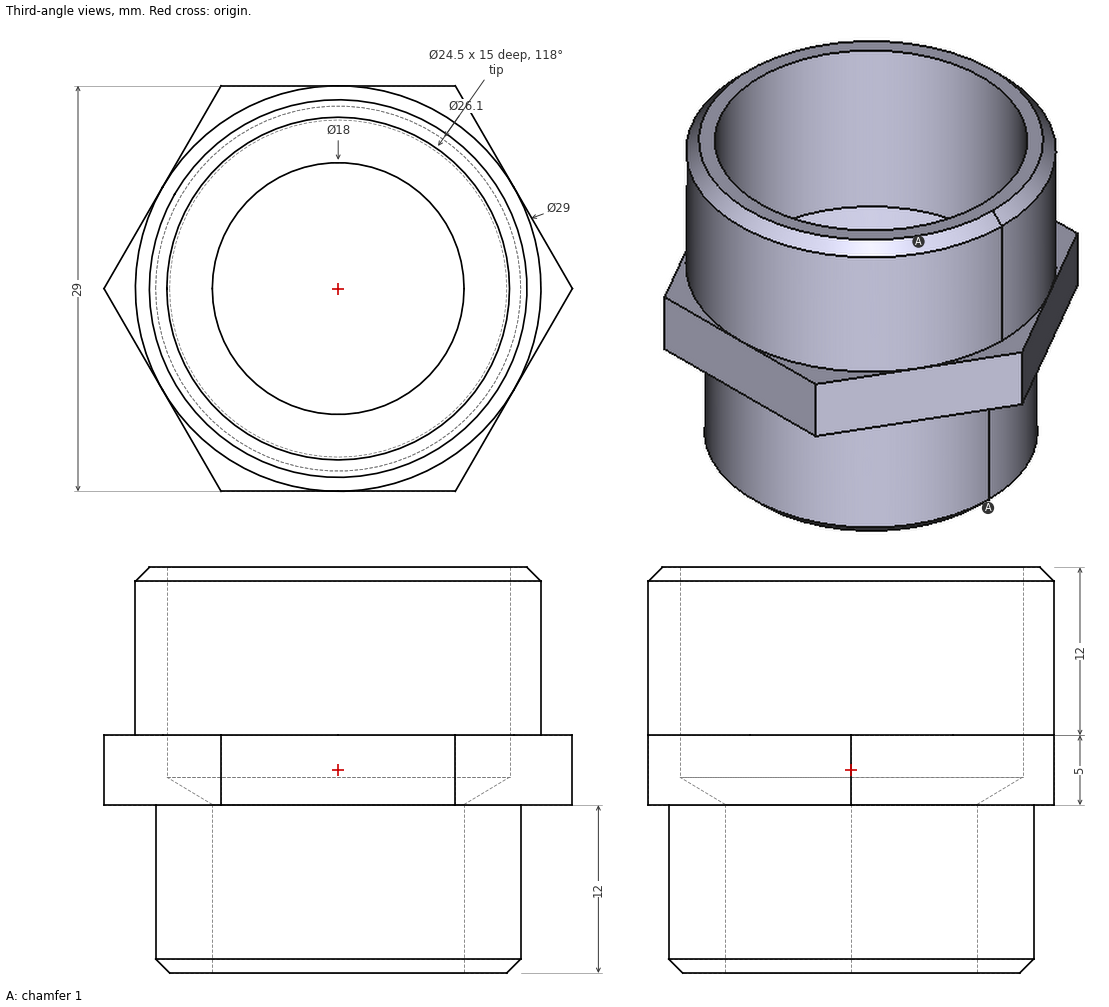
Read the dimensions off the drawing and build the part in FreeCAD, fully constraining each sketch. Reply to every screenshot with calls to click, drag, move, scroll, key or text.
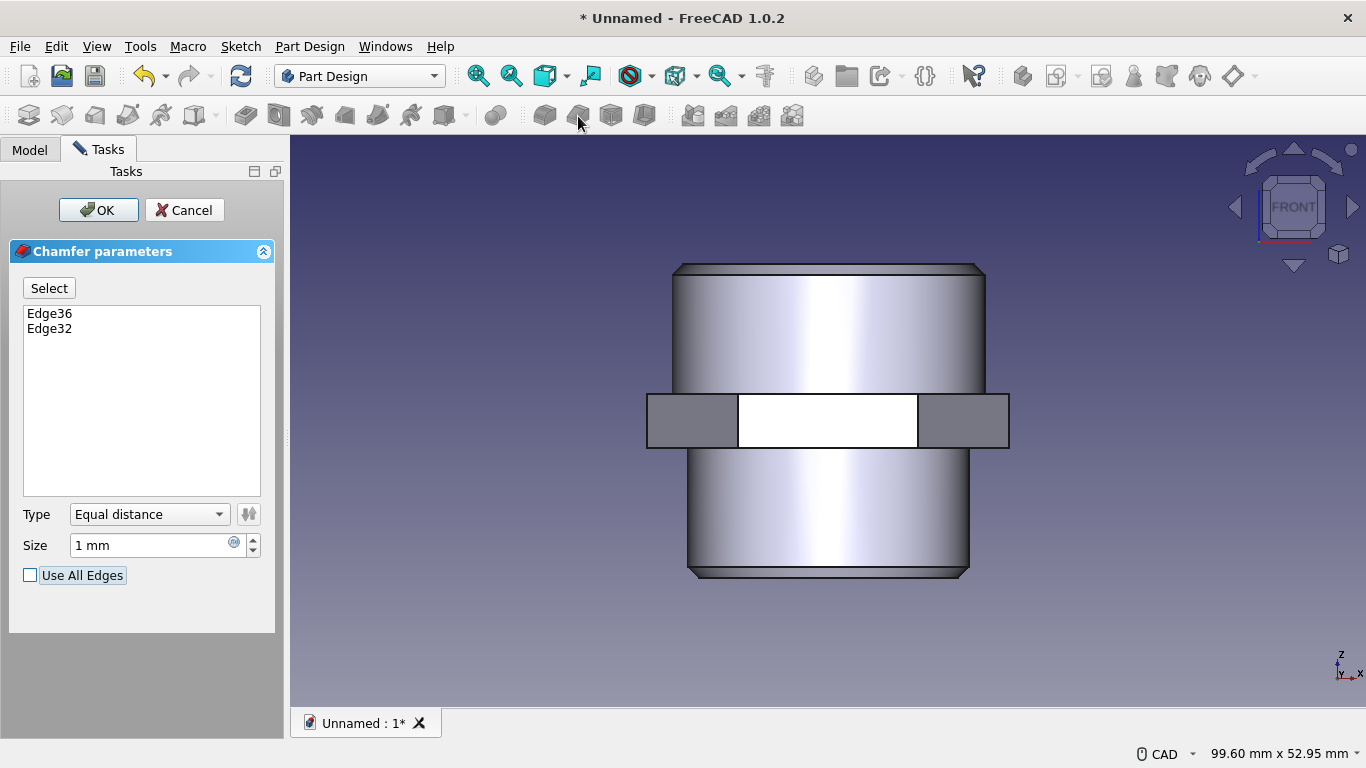
click(99, 210)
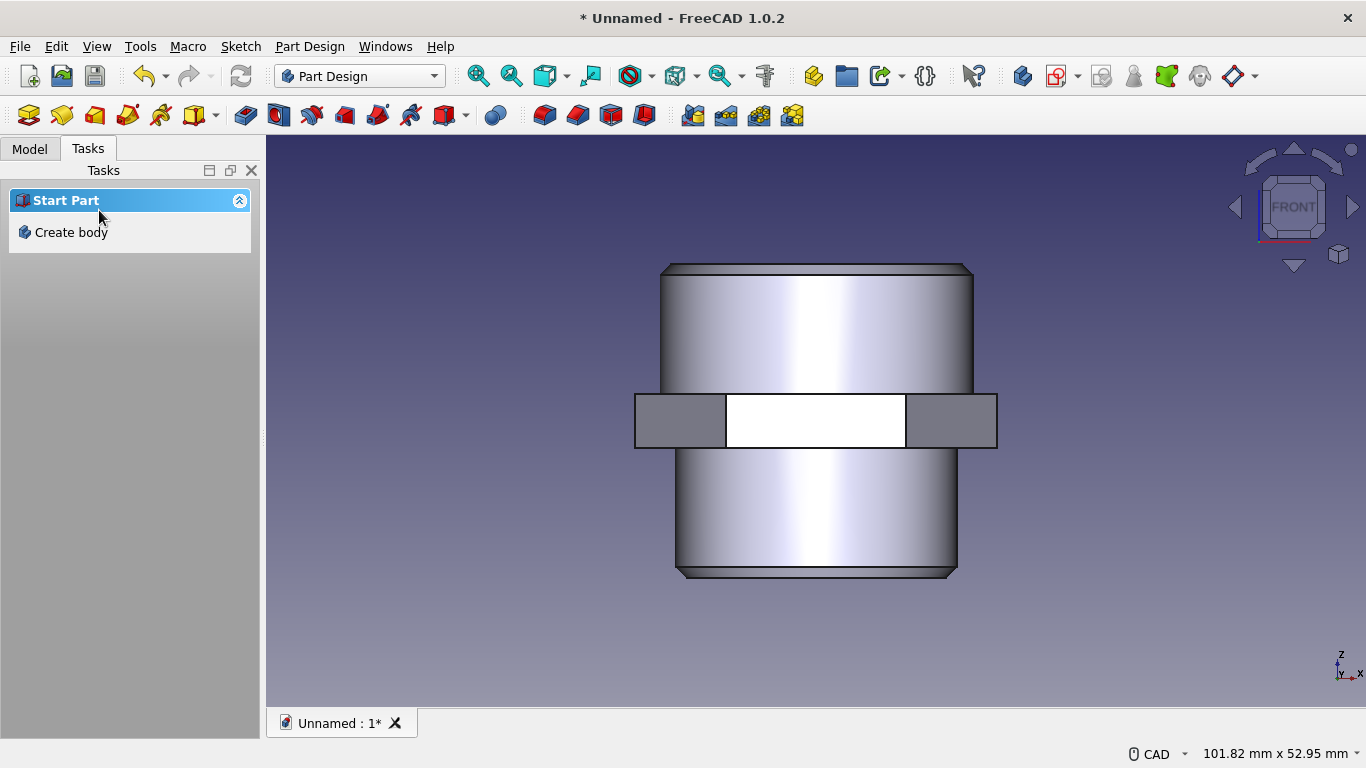
key(0)